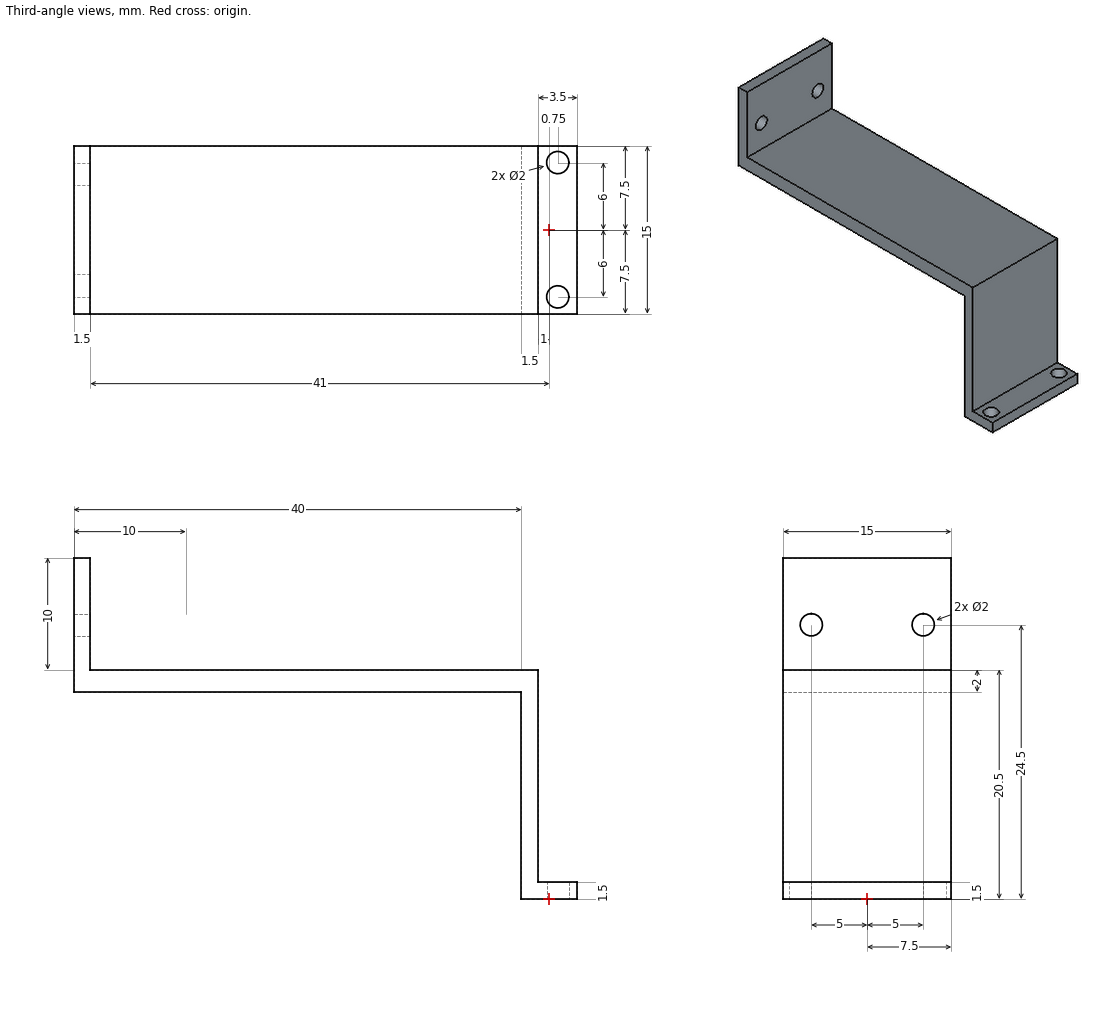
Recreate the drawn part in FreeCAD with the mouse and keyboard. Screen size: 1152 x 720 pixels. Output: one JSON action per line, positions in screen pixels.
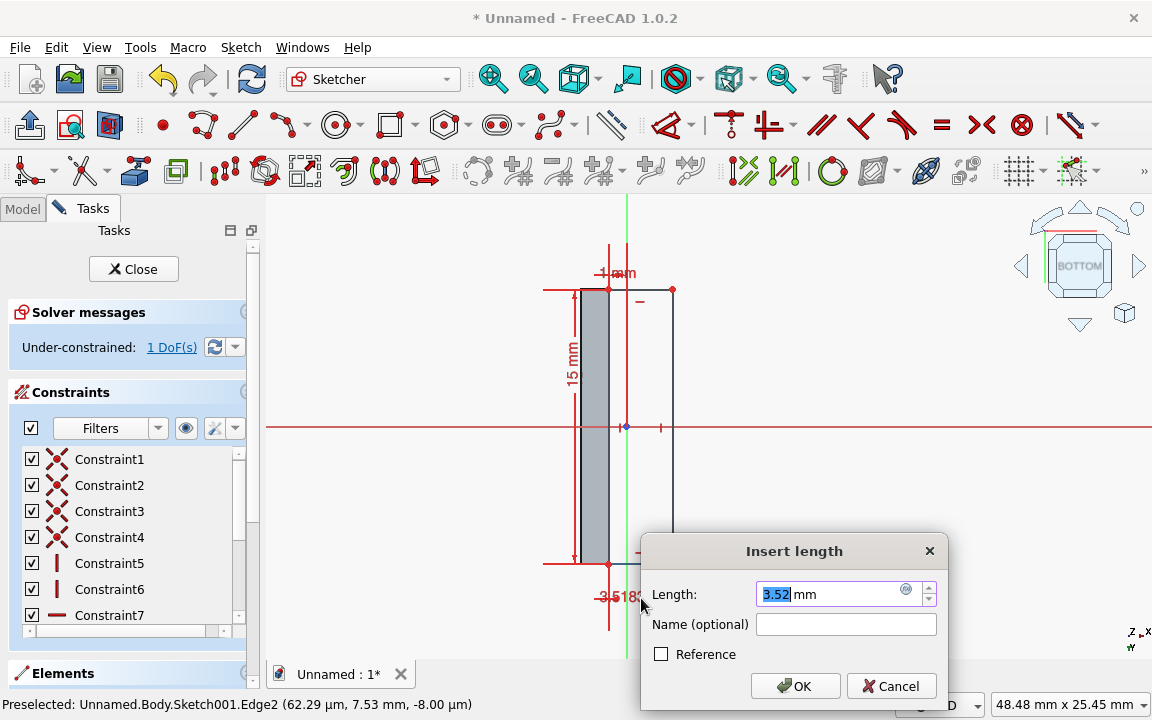
{"action": "type", "text": "3.5"}
{"action": "key", "text": "Return"}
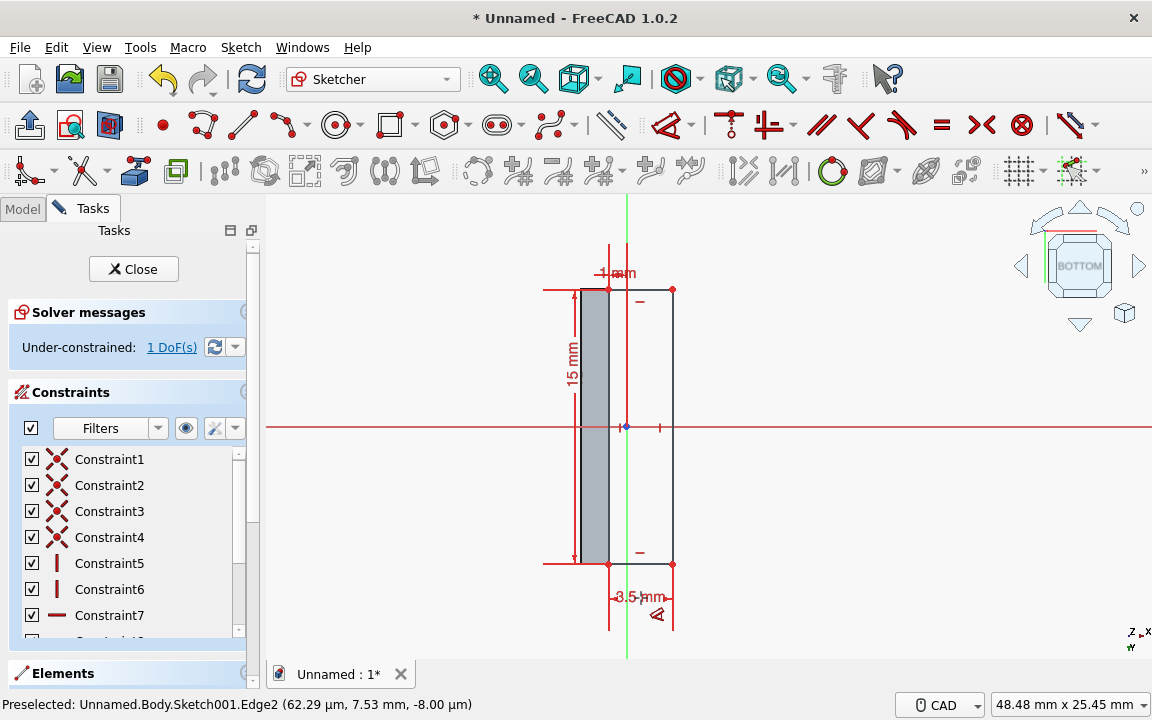
{"action": "left_click", "coordinate": [609, 290]}
{"action": "left_click", "coordinate": [575, 327]}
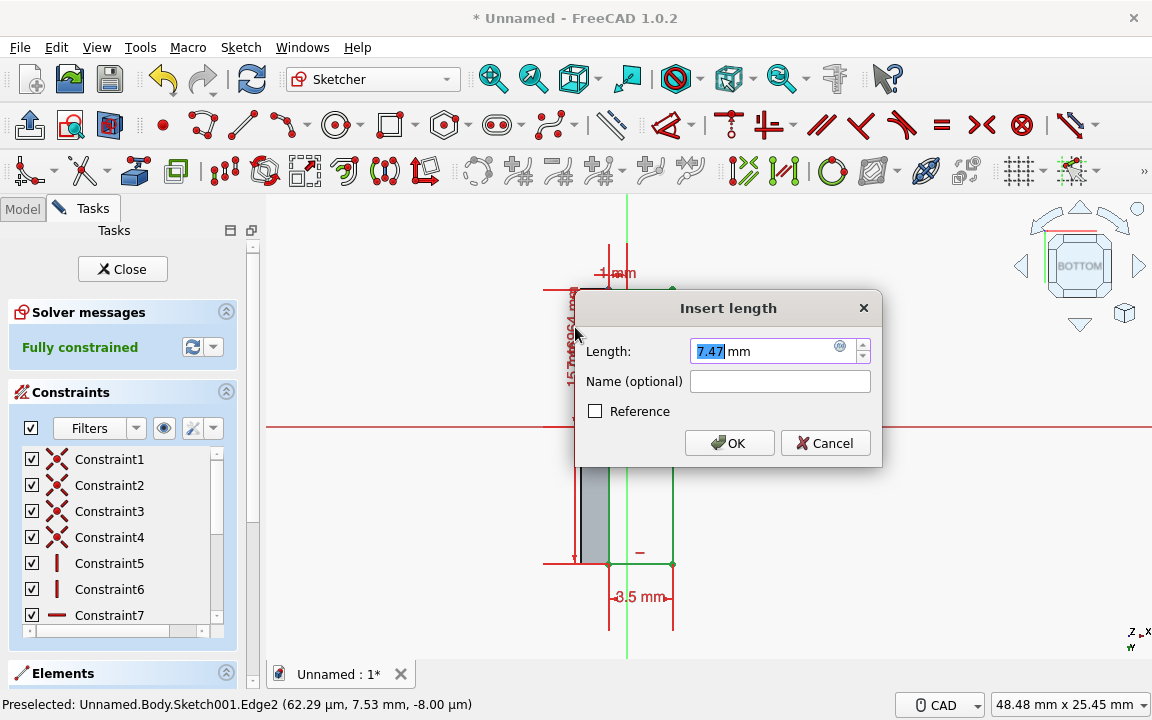
{"action": "type", "text": "7.5"}
{"action": "key", "text": "Return"}
{"action": "key", "text": "Escape"}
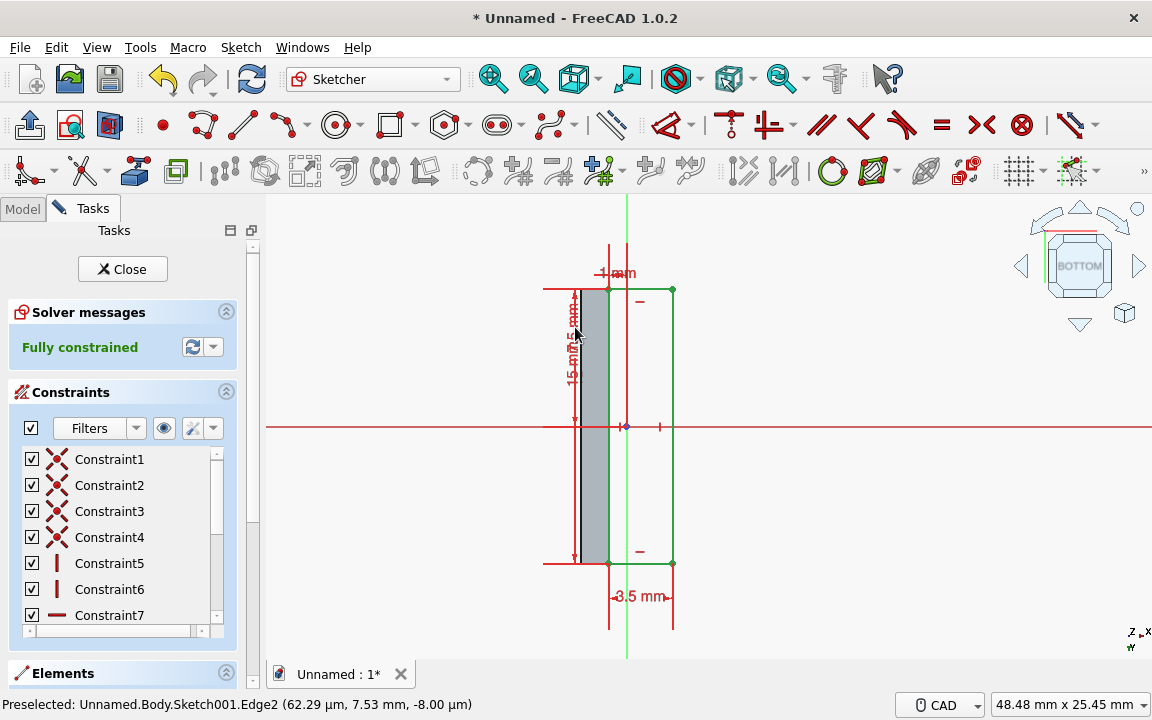
{"action": "left_click", "coordinate": [123, 269]}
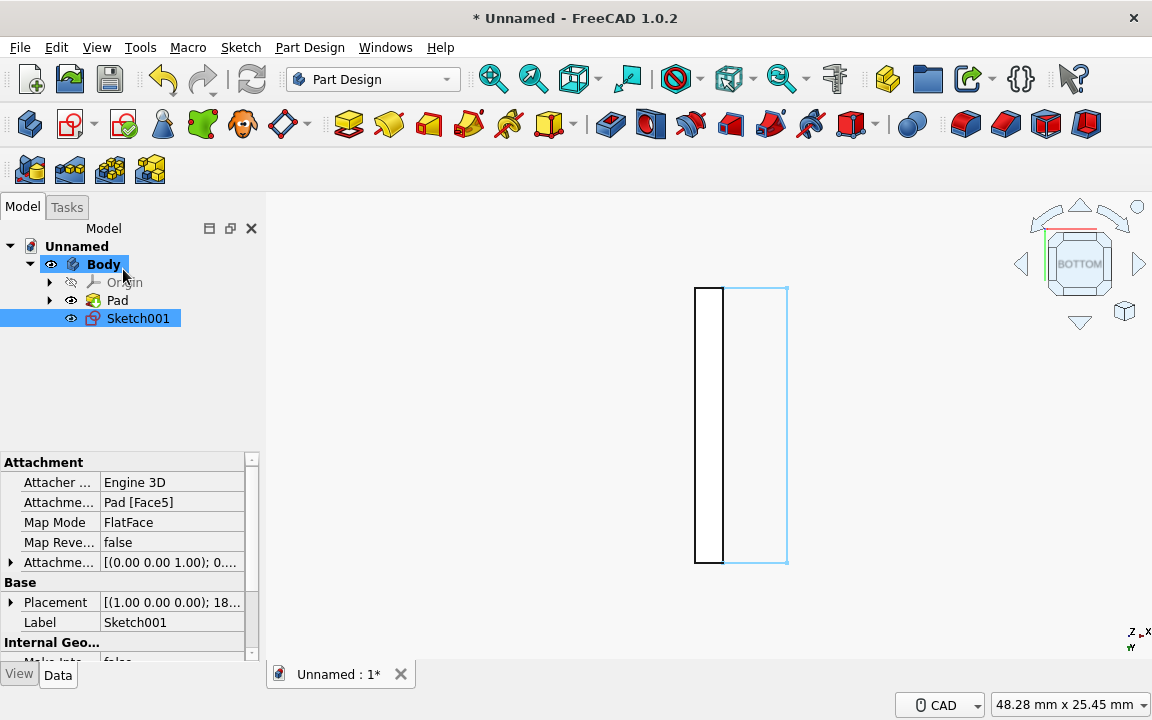
{"action": "left_click", "coordinate": [350, 124]}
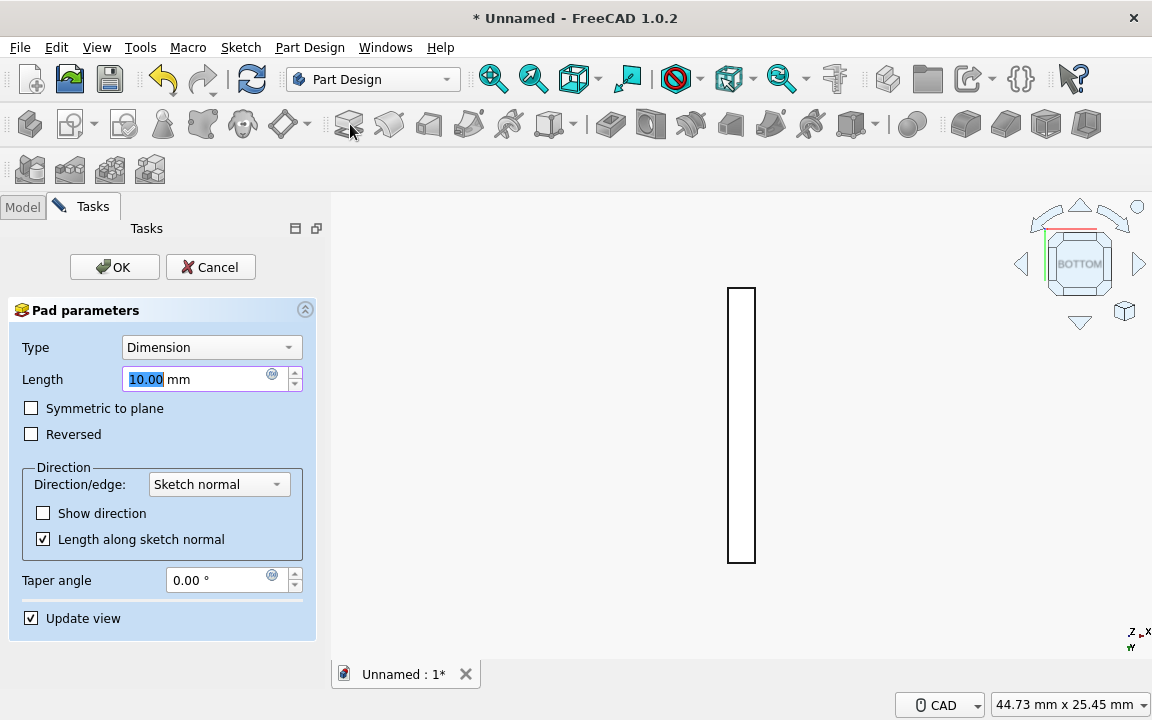
{"action": "type", "text": "1.5"}
{"action": "key", "text": "Tab"}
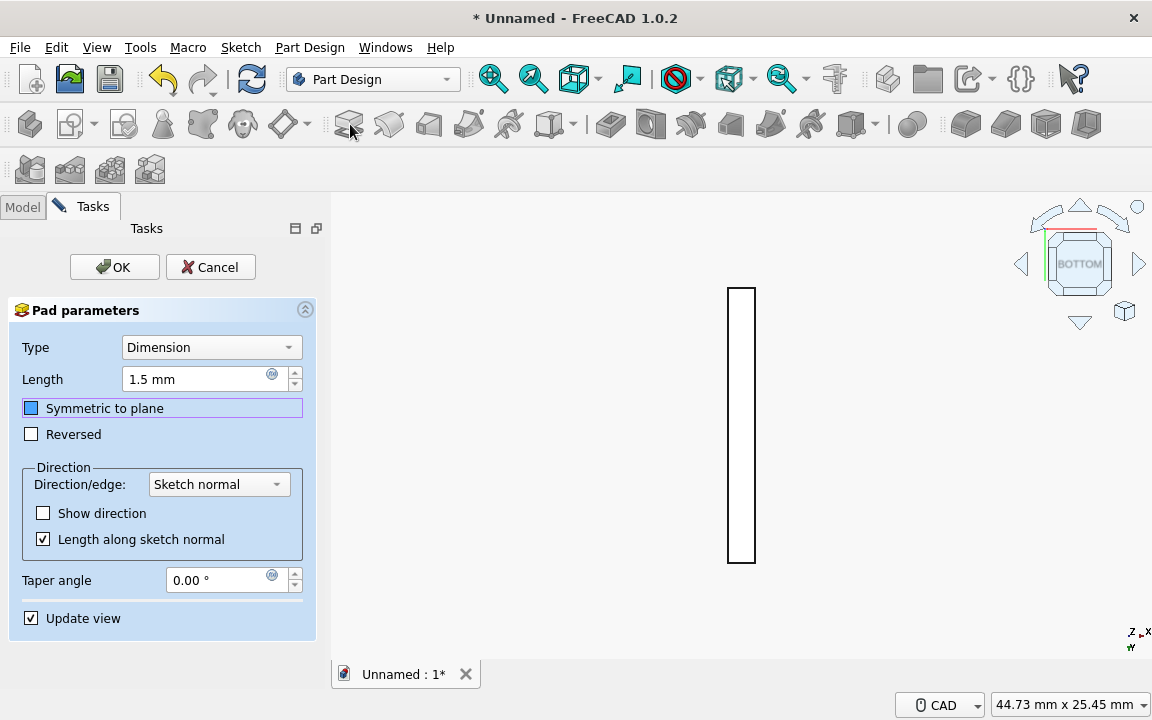
{"action": "left_click", "coordinate": [30, 434]}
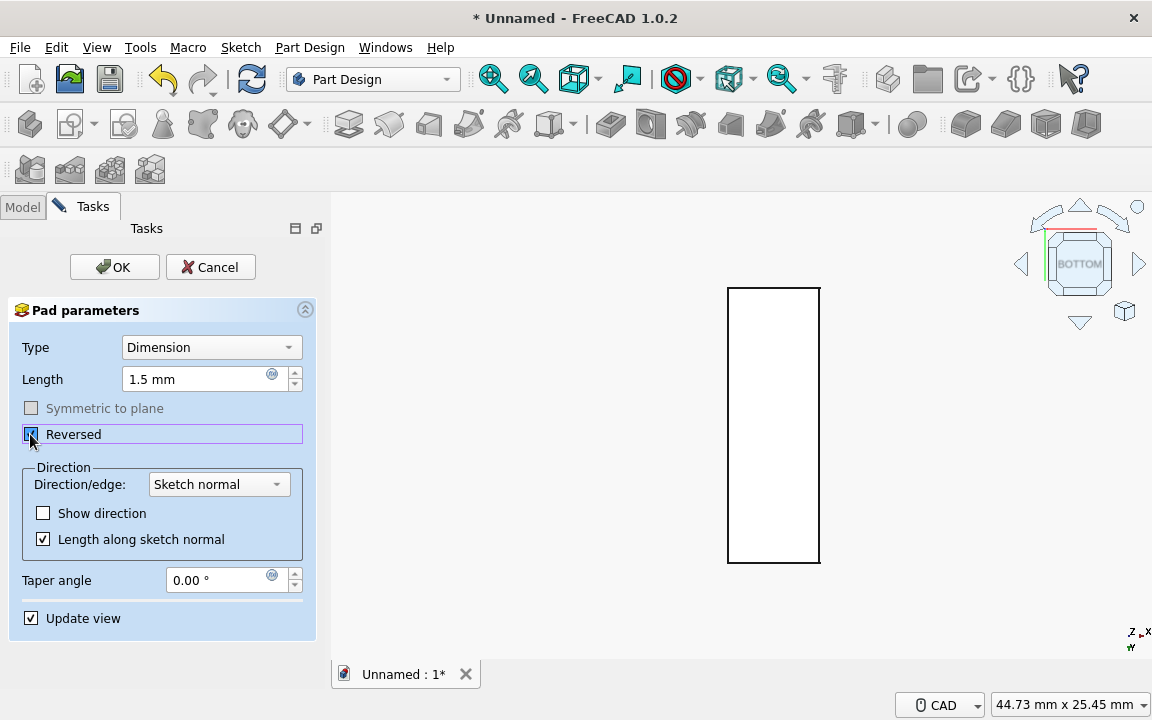
{"action": "left_click", "coordinate": [115, 267]}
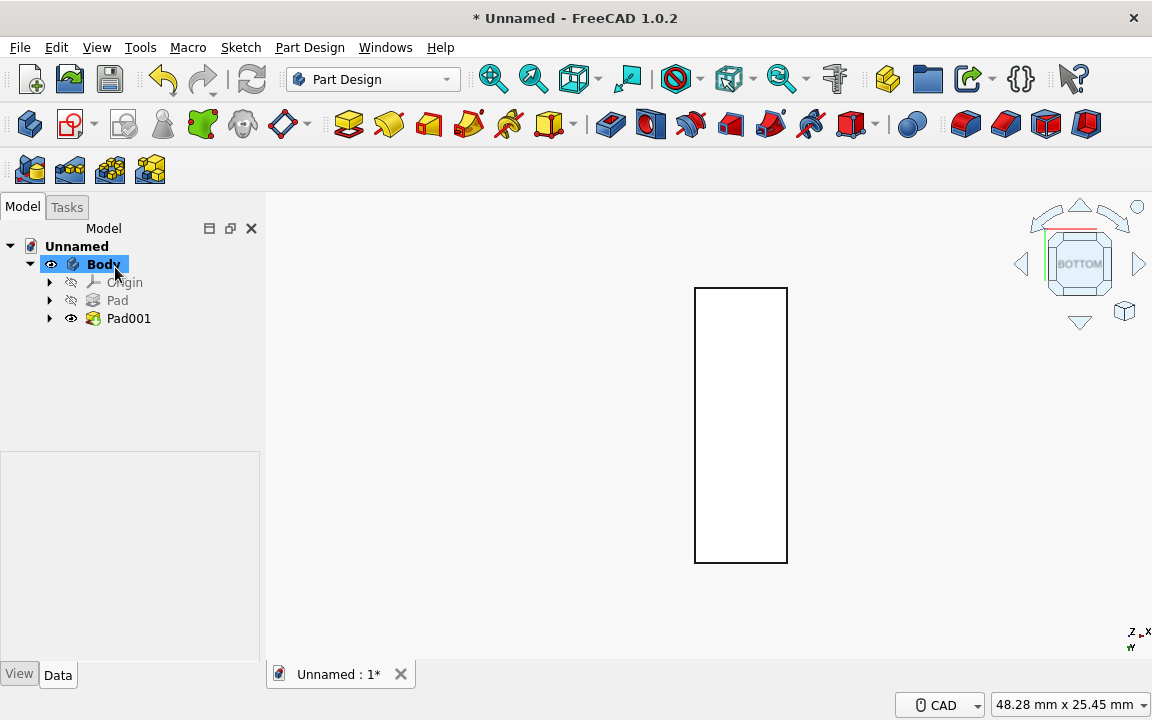
{"action": "key", "text": "0"}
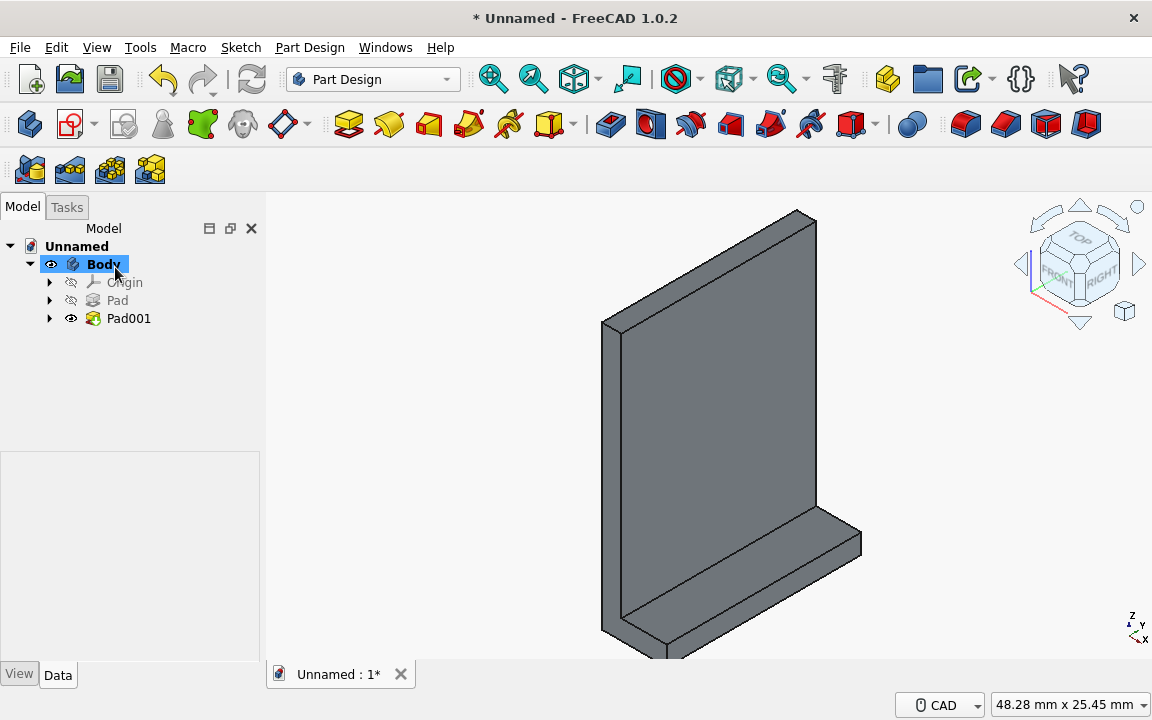
{"action": "left_click", "coordinate": [494, 80]}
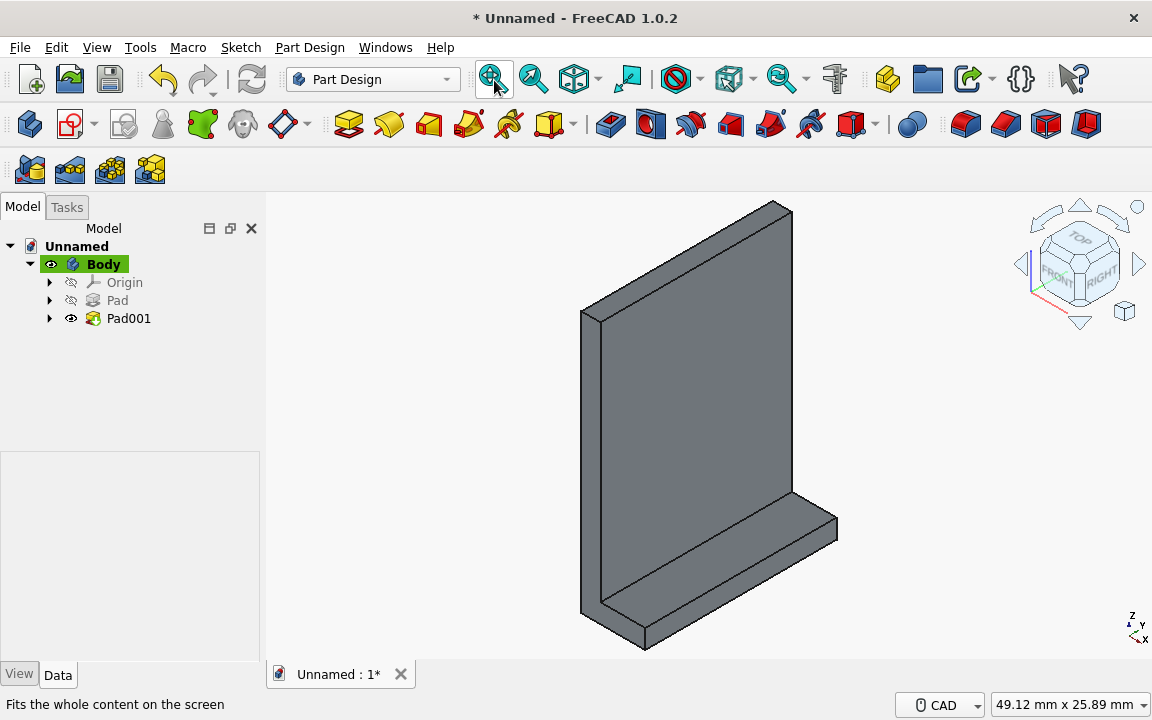
{"action": "left_click", "coordinate": [773, 527]}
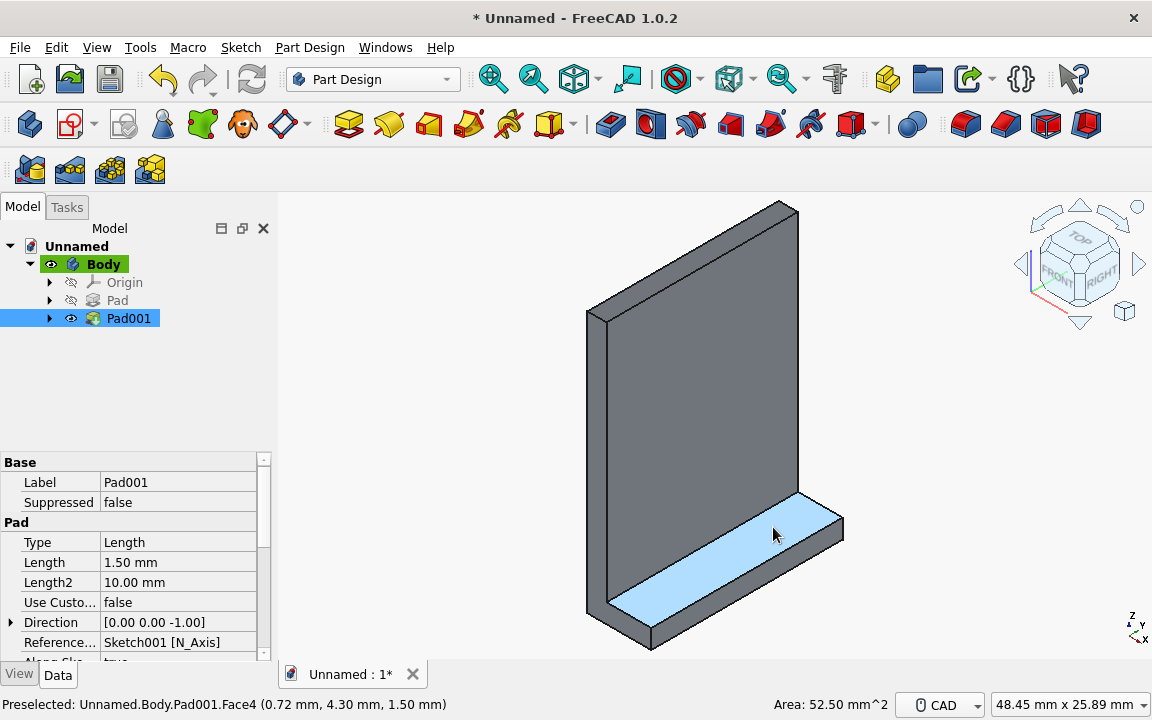
{"action": "left_click", "coordinate": [70, 124]}